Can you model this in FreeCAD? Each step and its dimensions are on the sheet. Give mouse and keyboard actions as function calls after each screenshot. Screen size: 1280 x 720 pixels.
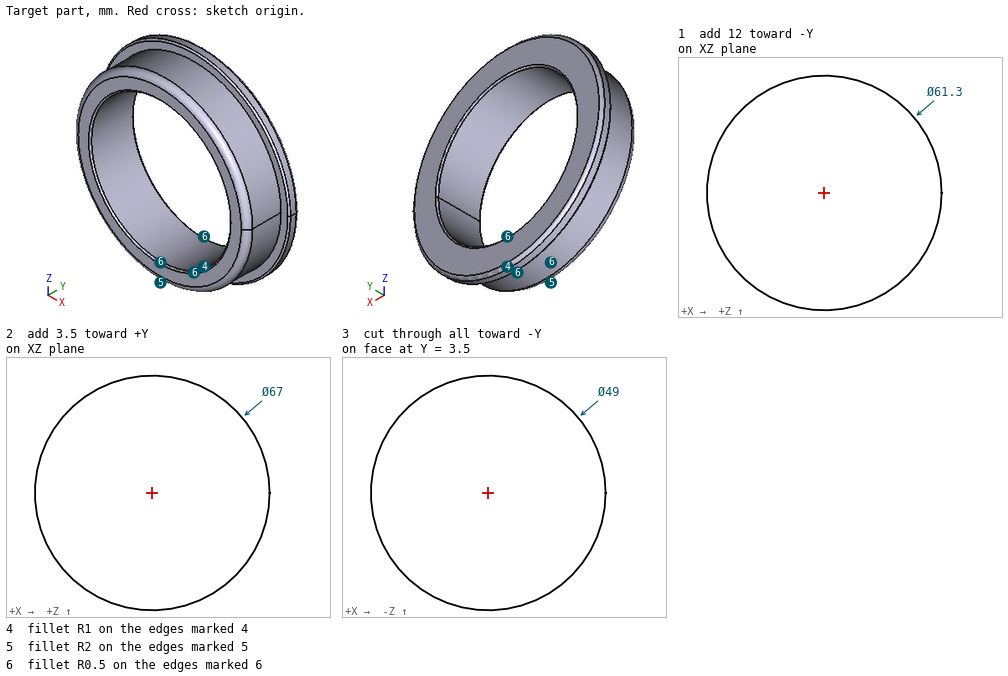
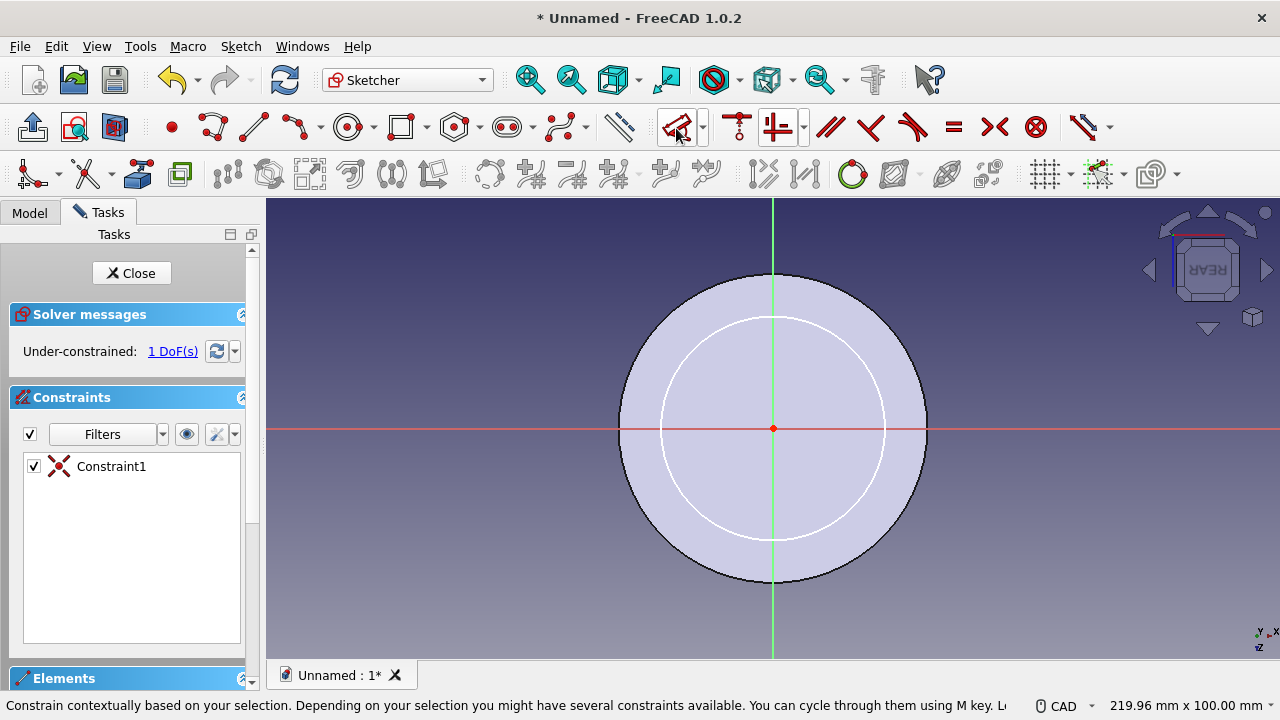
click(852, 349)
click(875, 326)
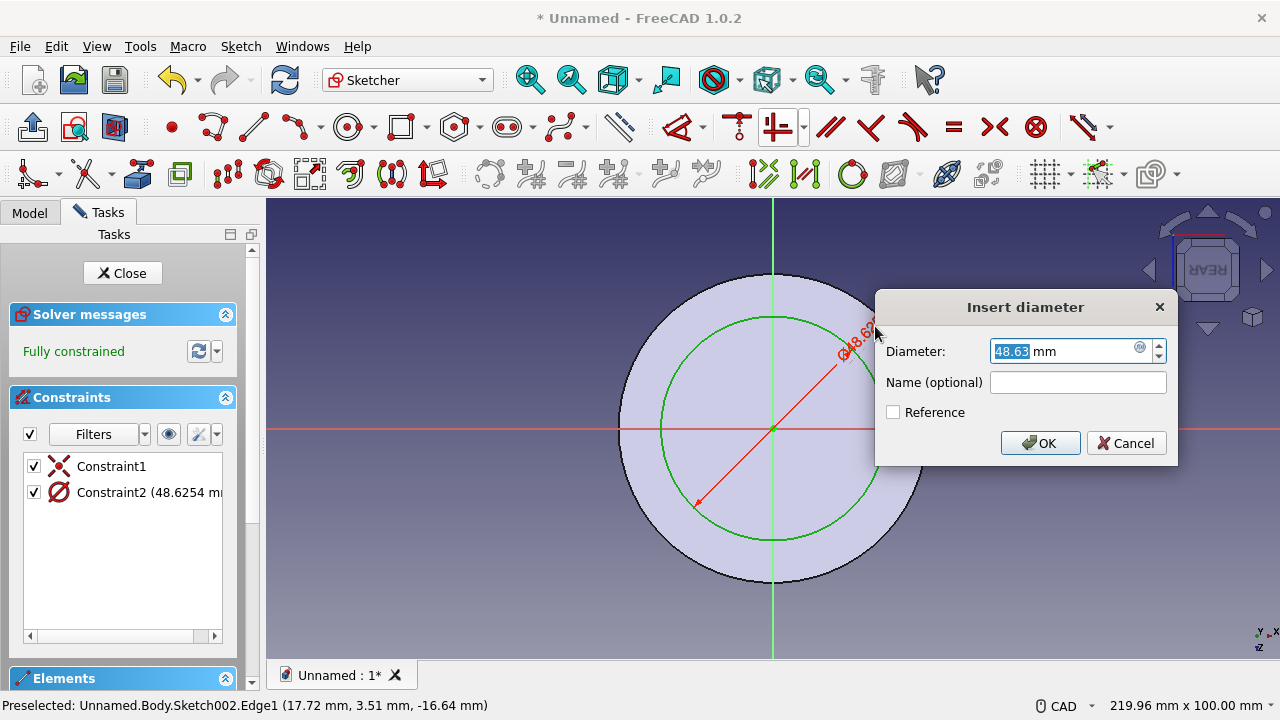
text(49)
key(Return)
key(Escape)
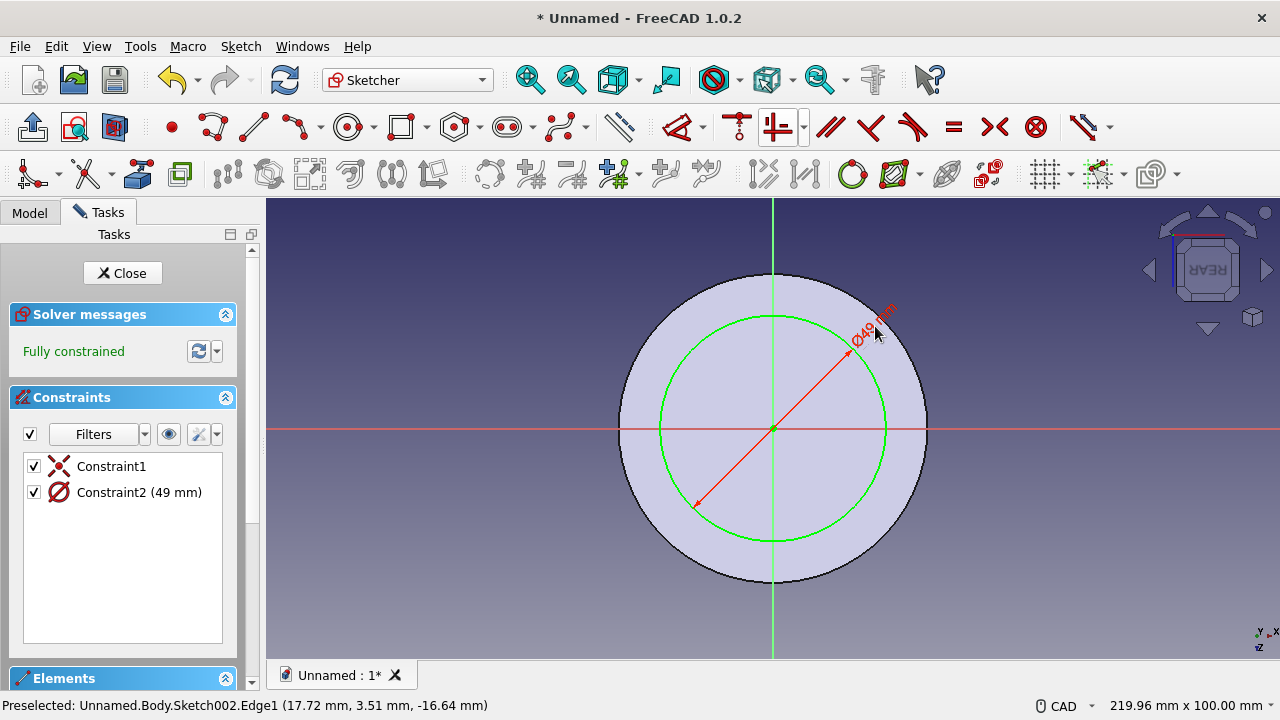
click(123, 273)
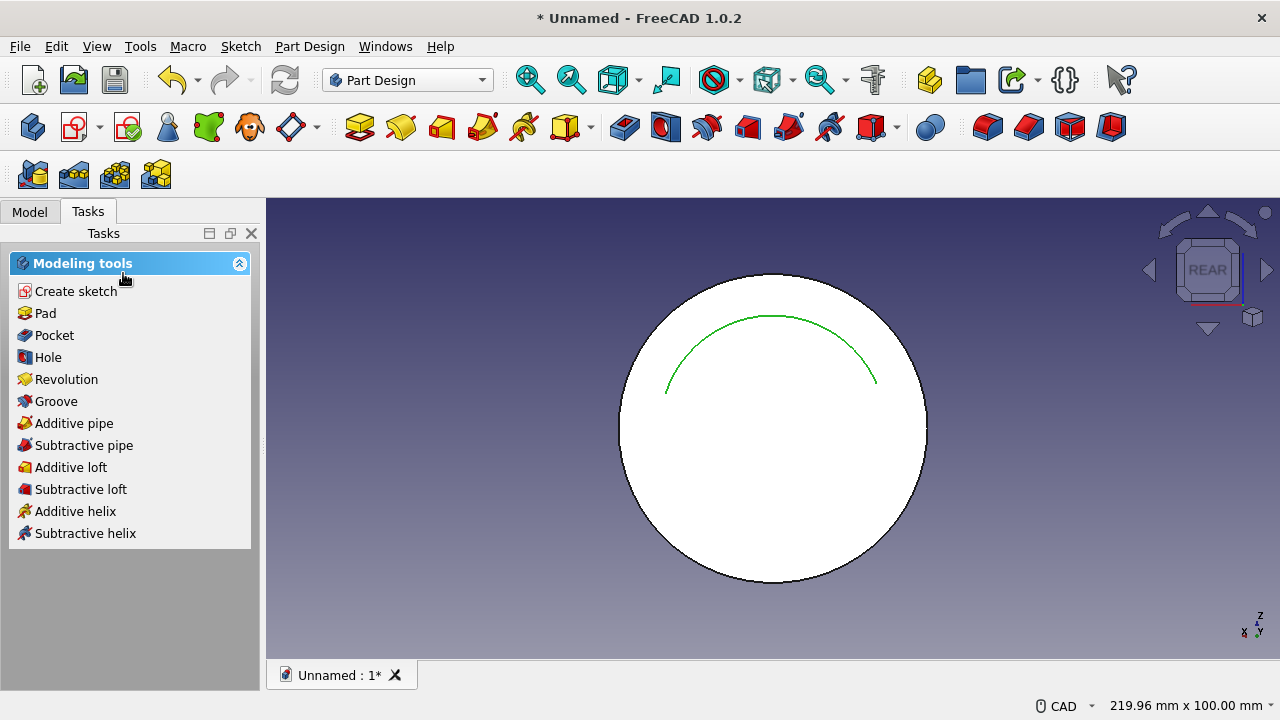
click(625, 128)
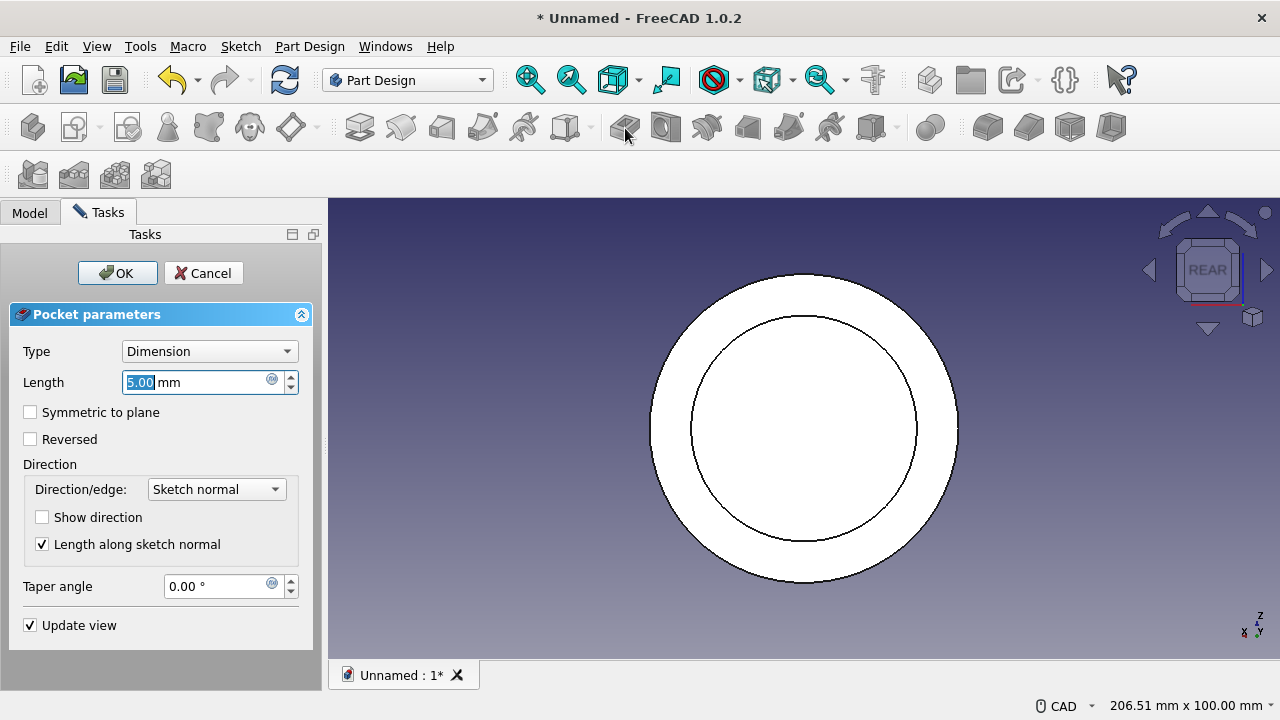
click(210, 352)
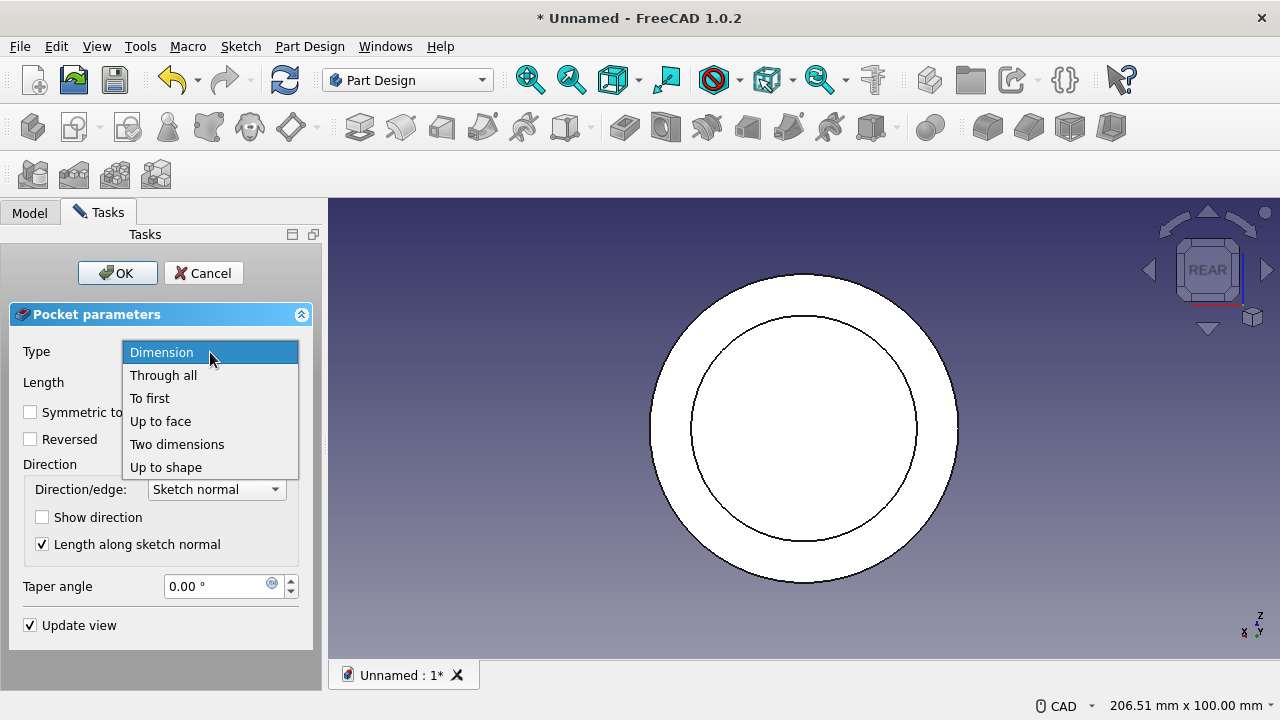
click(208, 376)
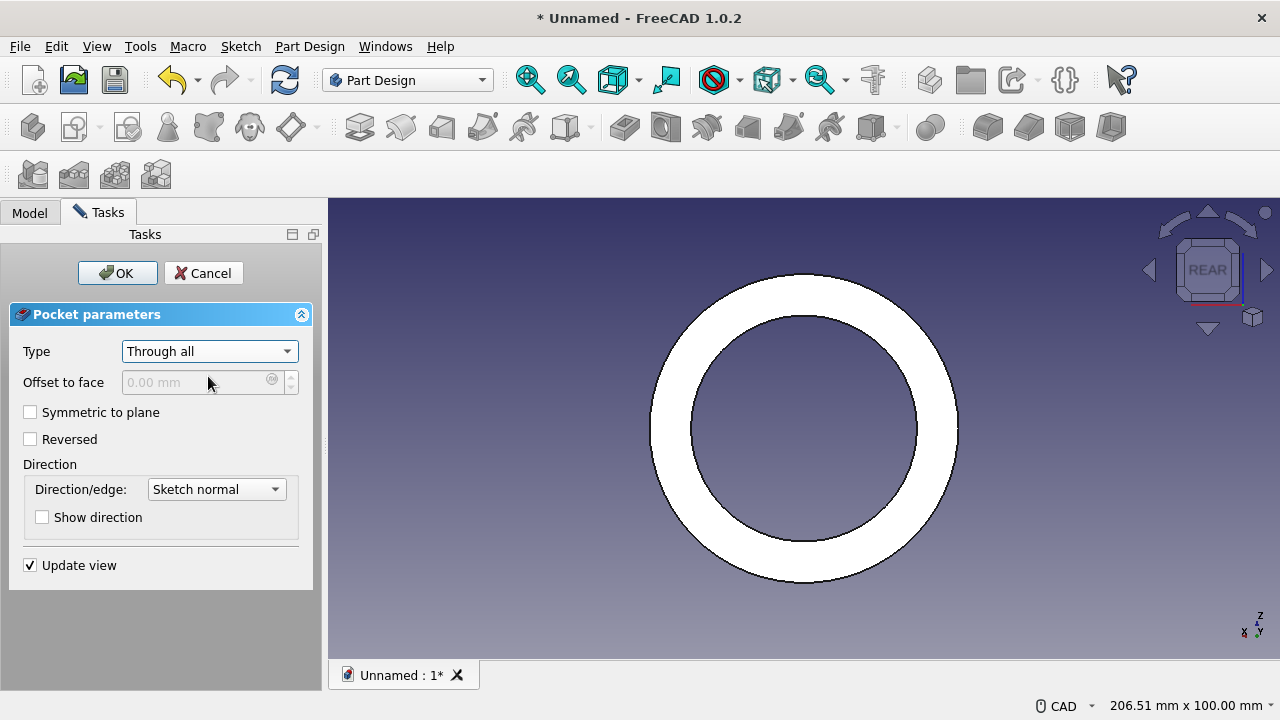
click(118, 273)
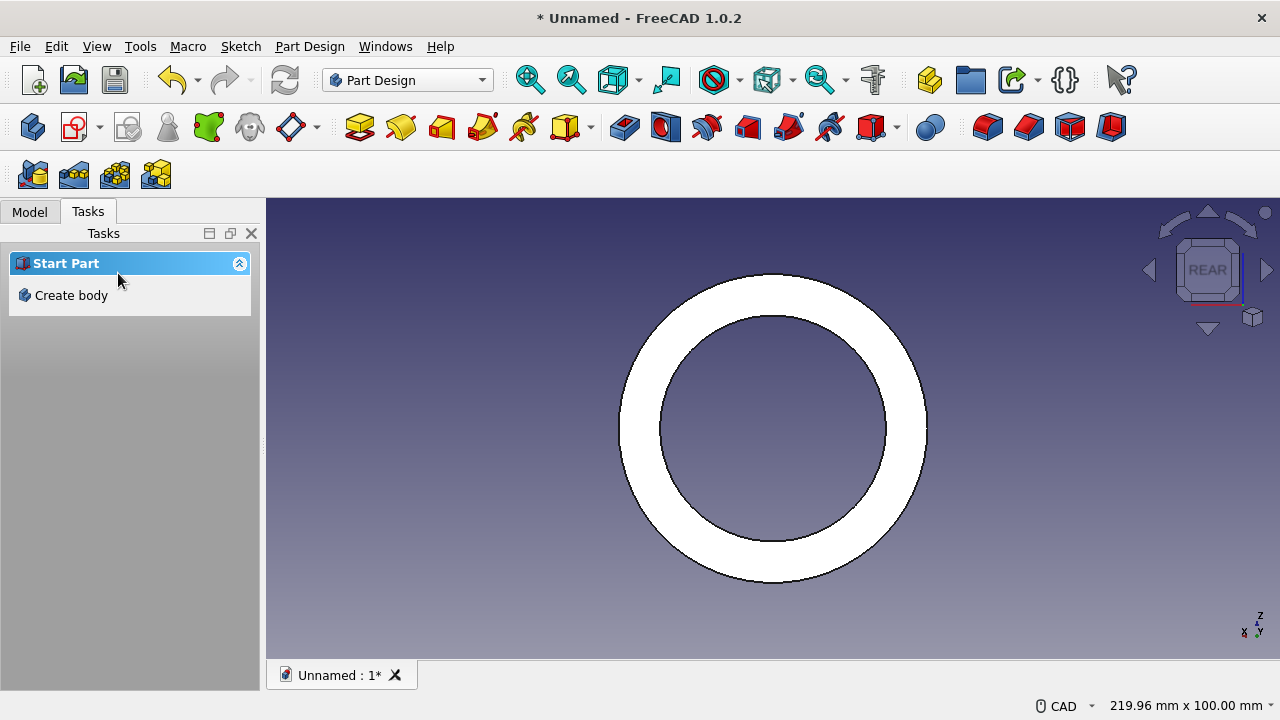
click(927, 428)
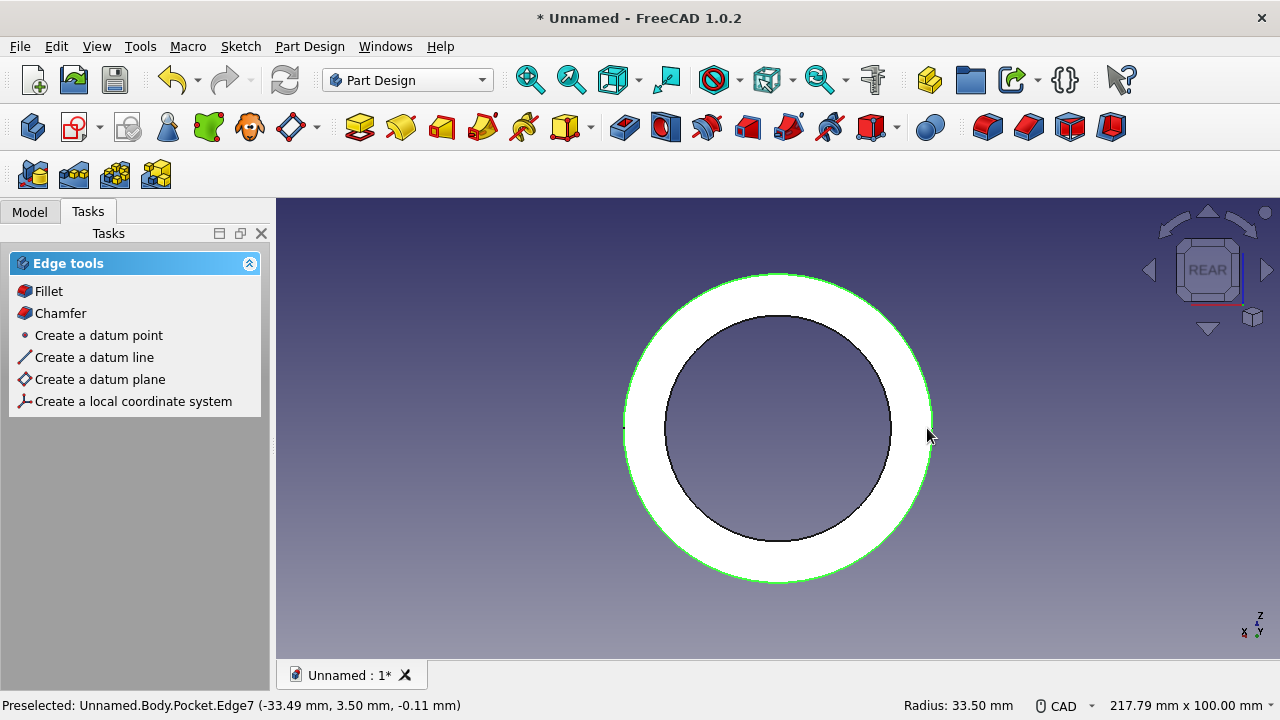
click(988, 128)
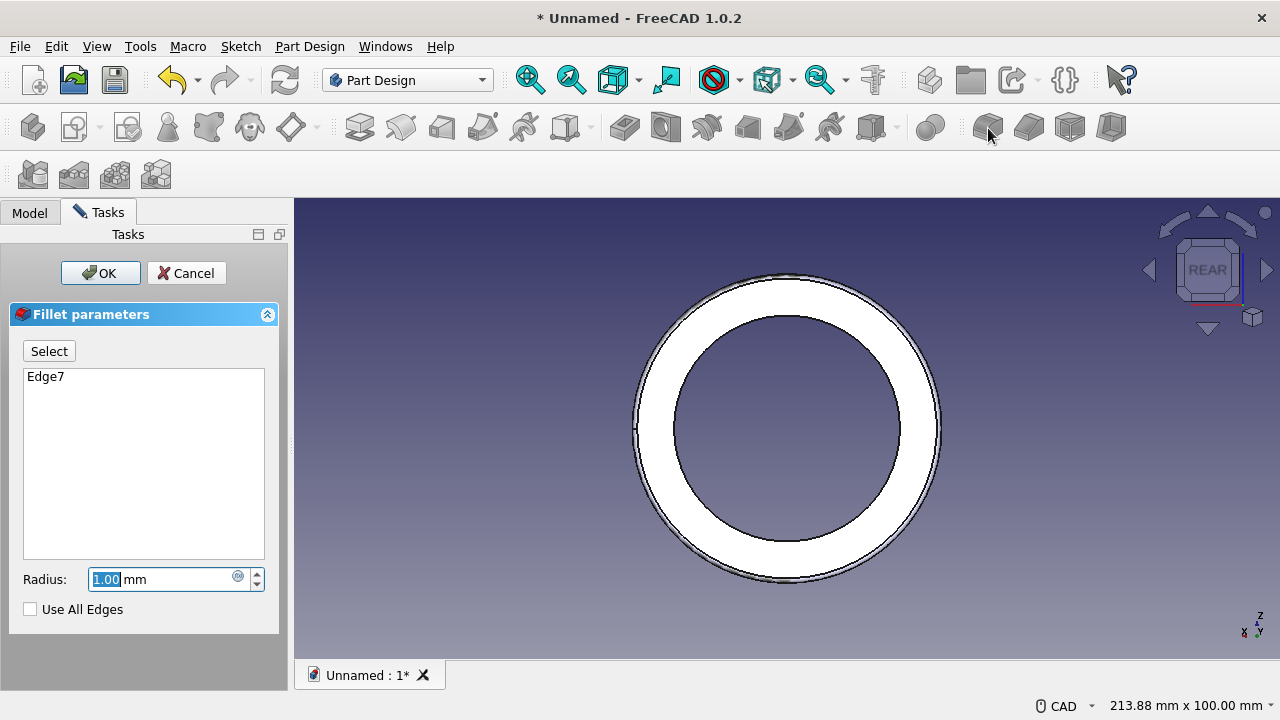
text(1)
key(Tab)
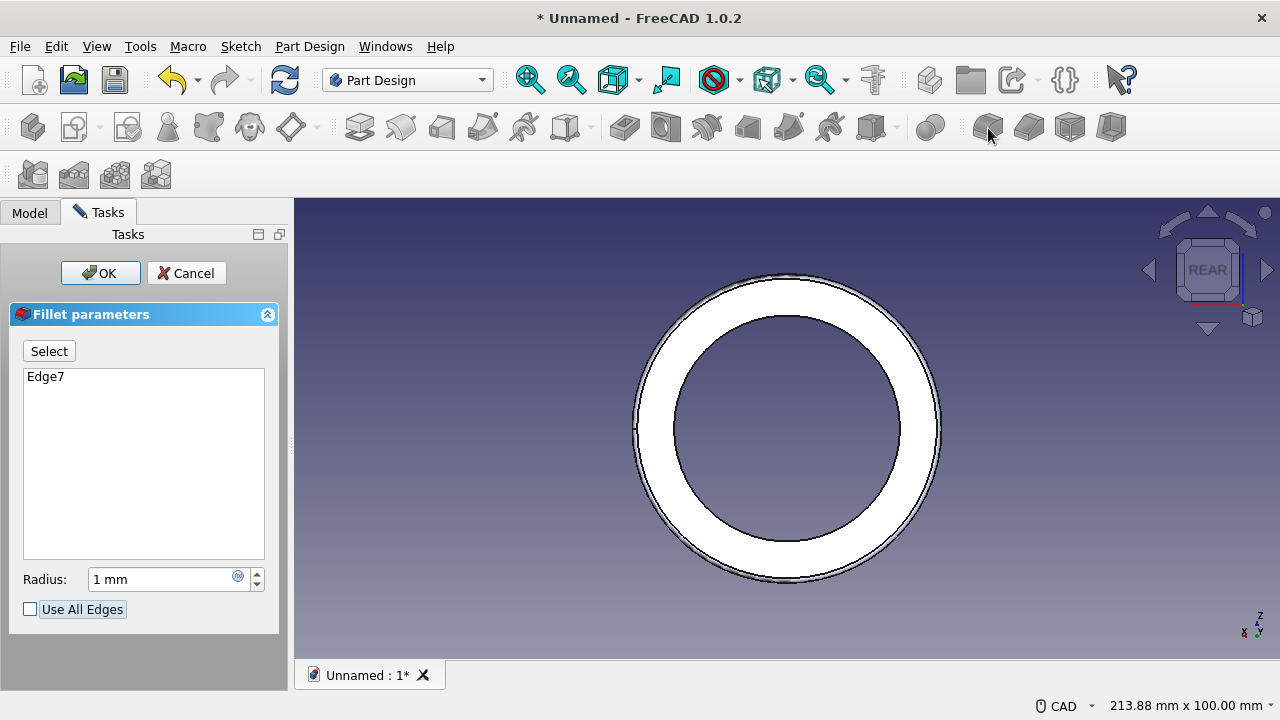
click(101, 273)